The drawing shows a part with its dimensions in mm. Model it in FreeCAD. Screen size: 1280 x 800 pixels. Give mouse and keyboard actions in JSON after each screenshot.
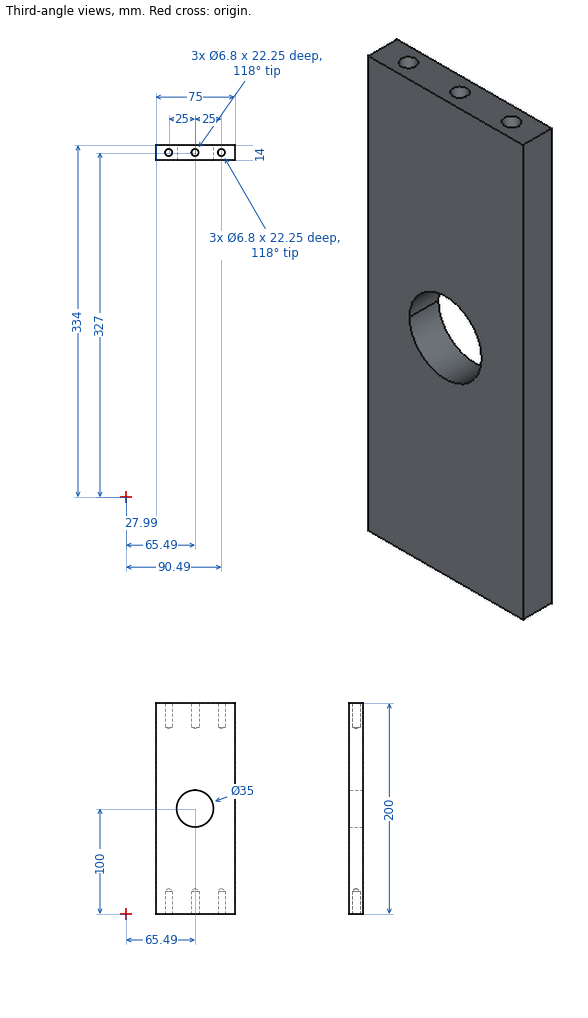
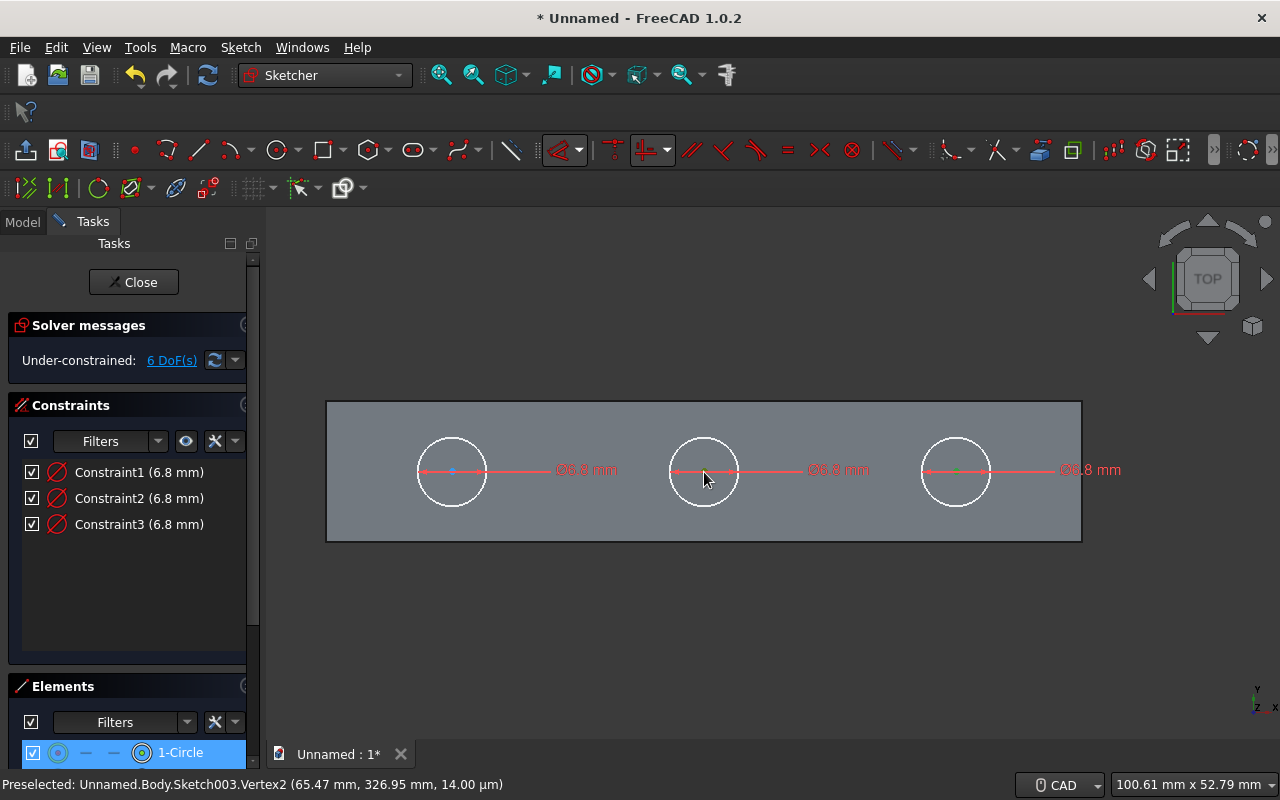
{"action": "key", "text": "h"}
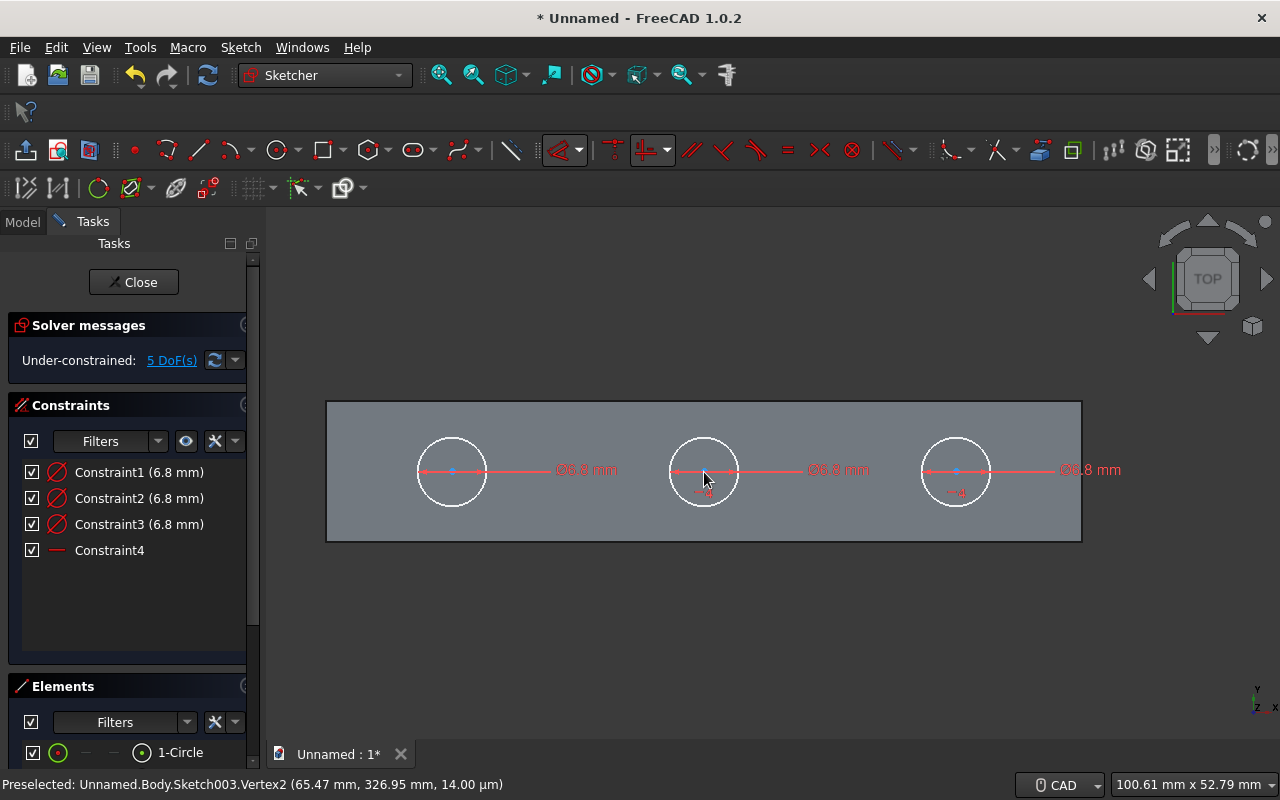
{"action": "left_click", "coordinate": [704, 472]}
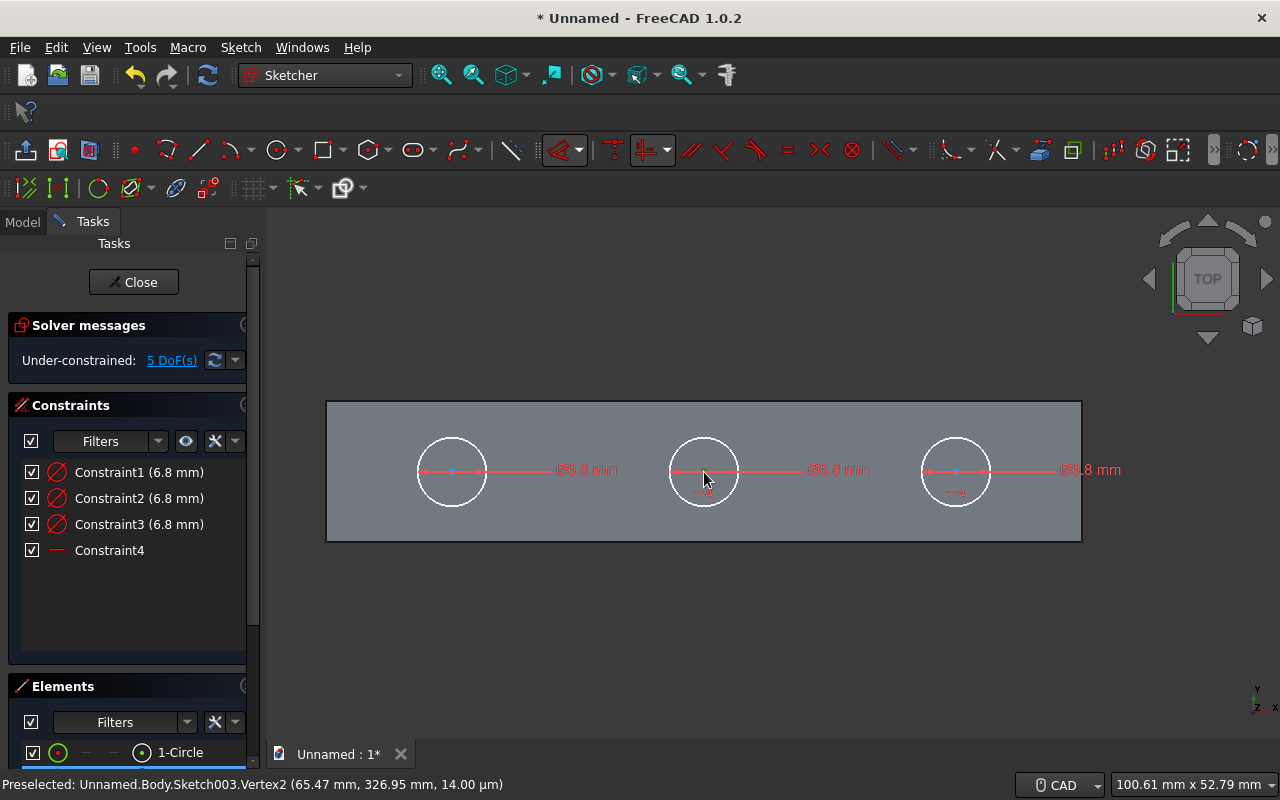
{"action": "left_click", "coordinate": [452, 472]}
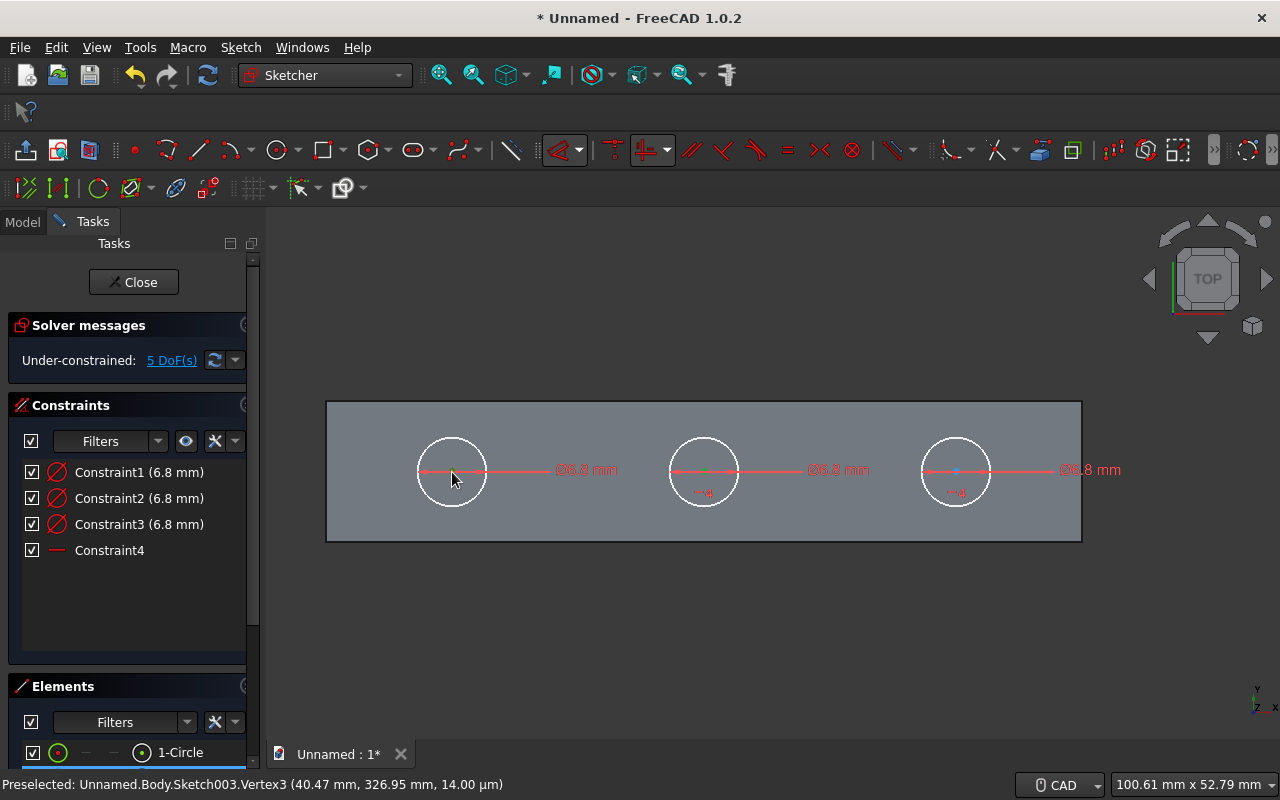
{"action": "left_click", "coordinate": [670, 150]}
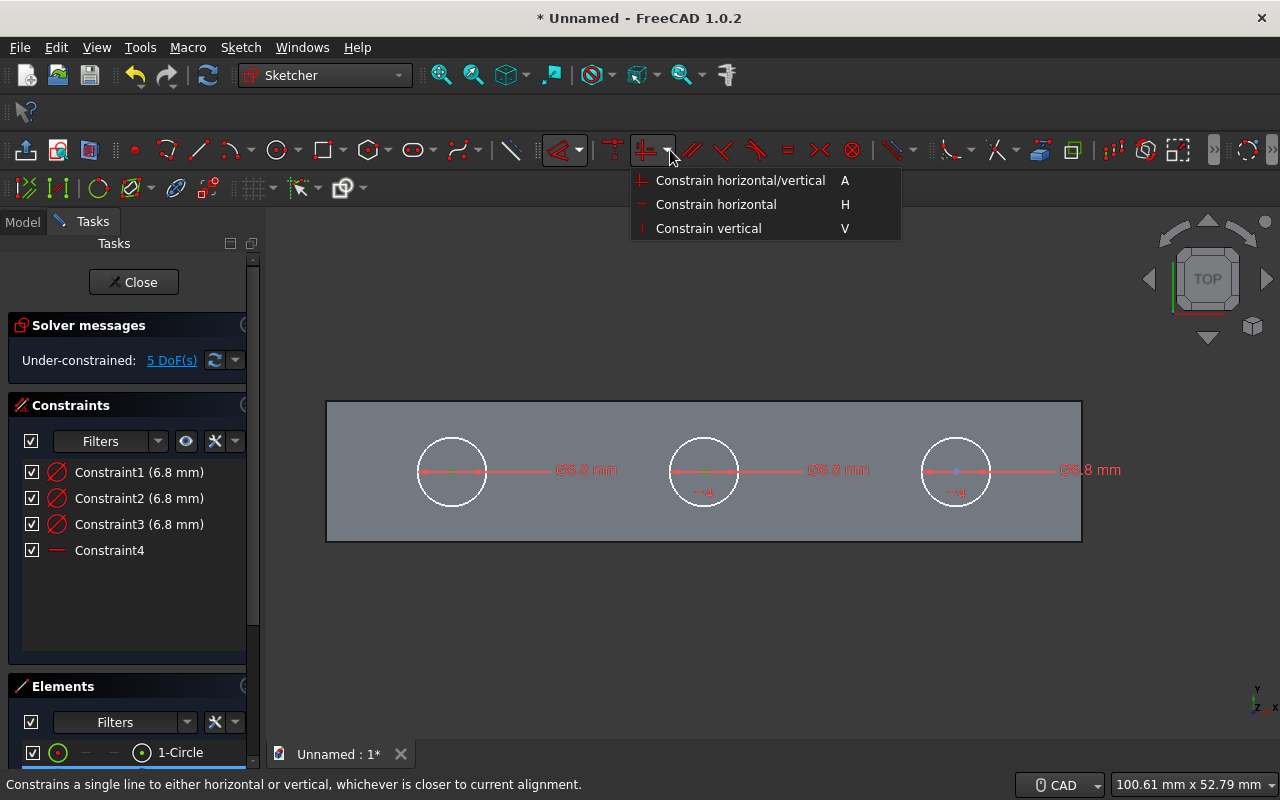
{"action": "left_click", "coordinate": [766, 204]}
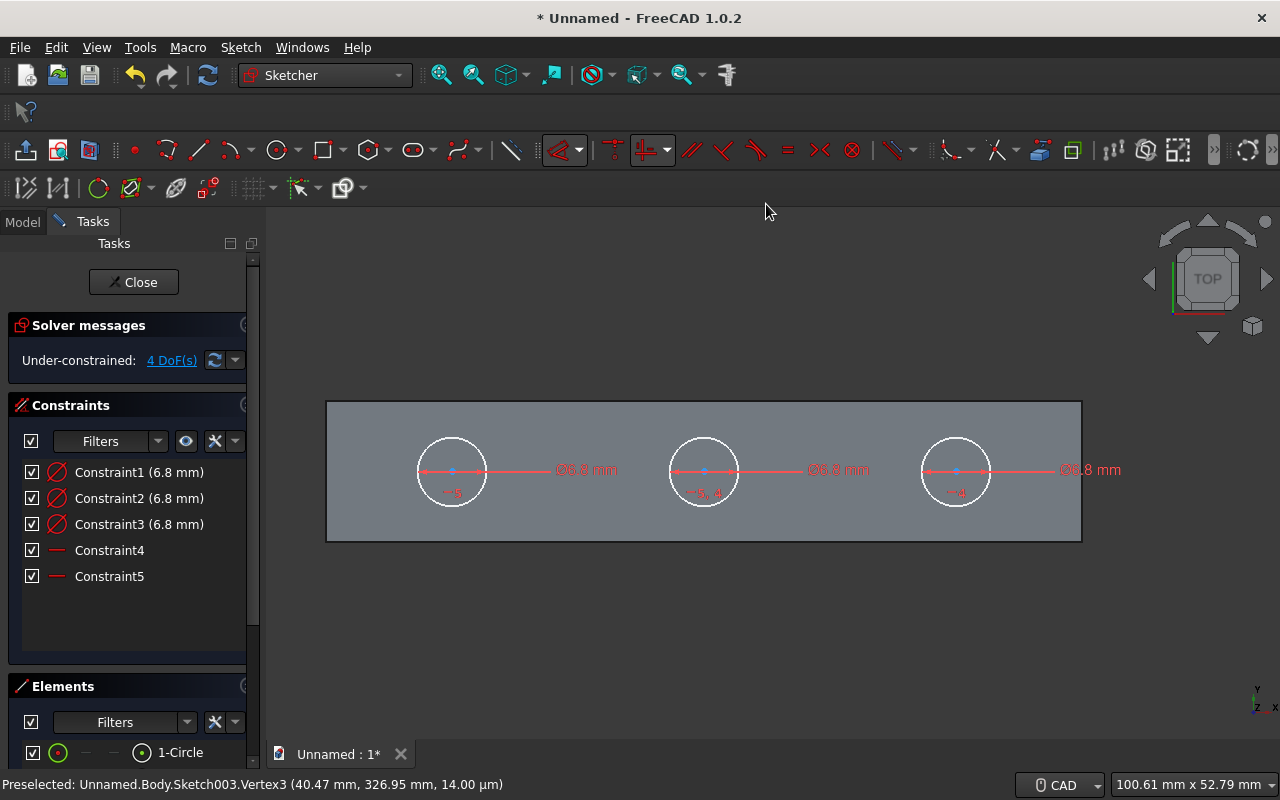
{"action": "left_click", "coordinate": [956, 472]}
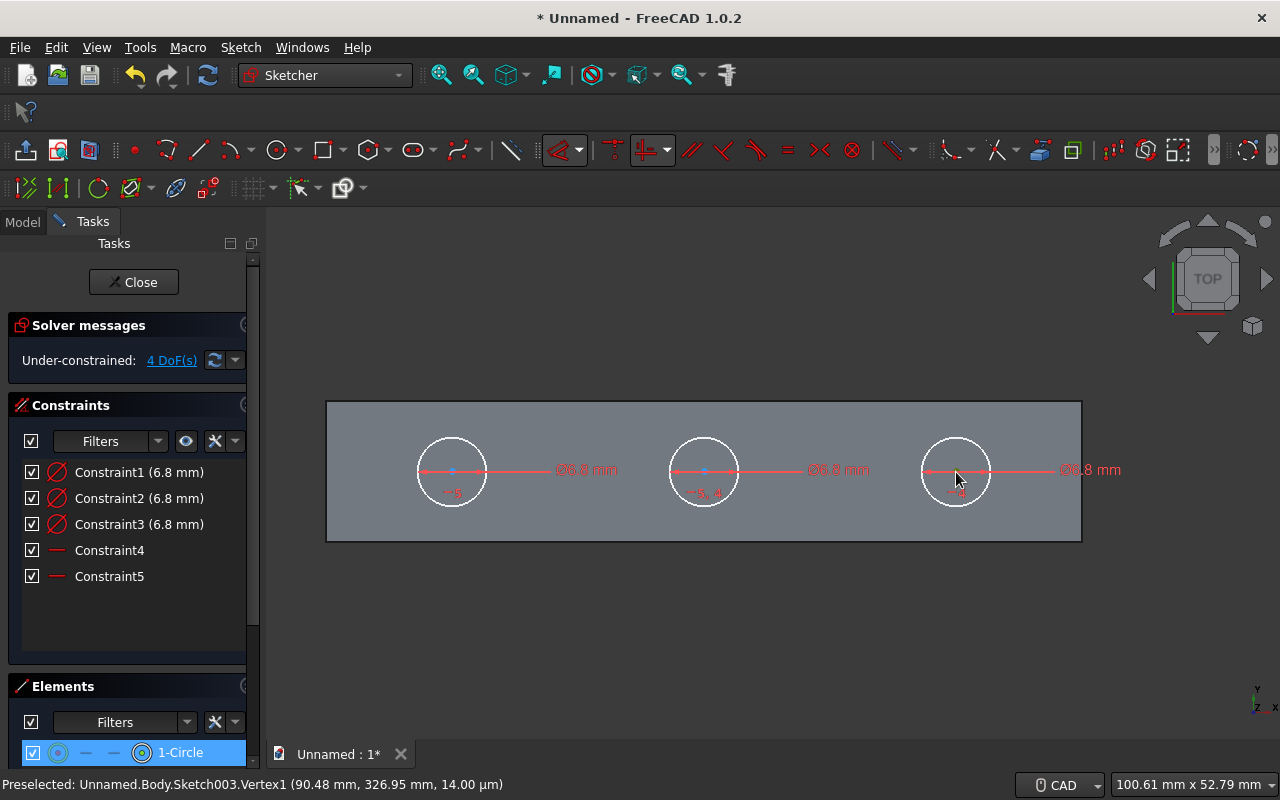
{"action": "left_click", "coordinate": [582, 150]}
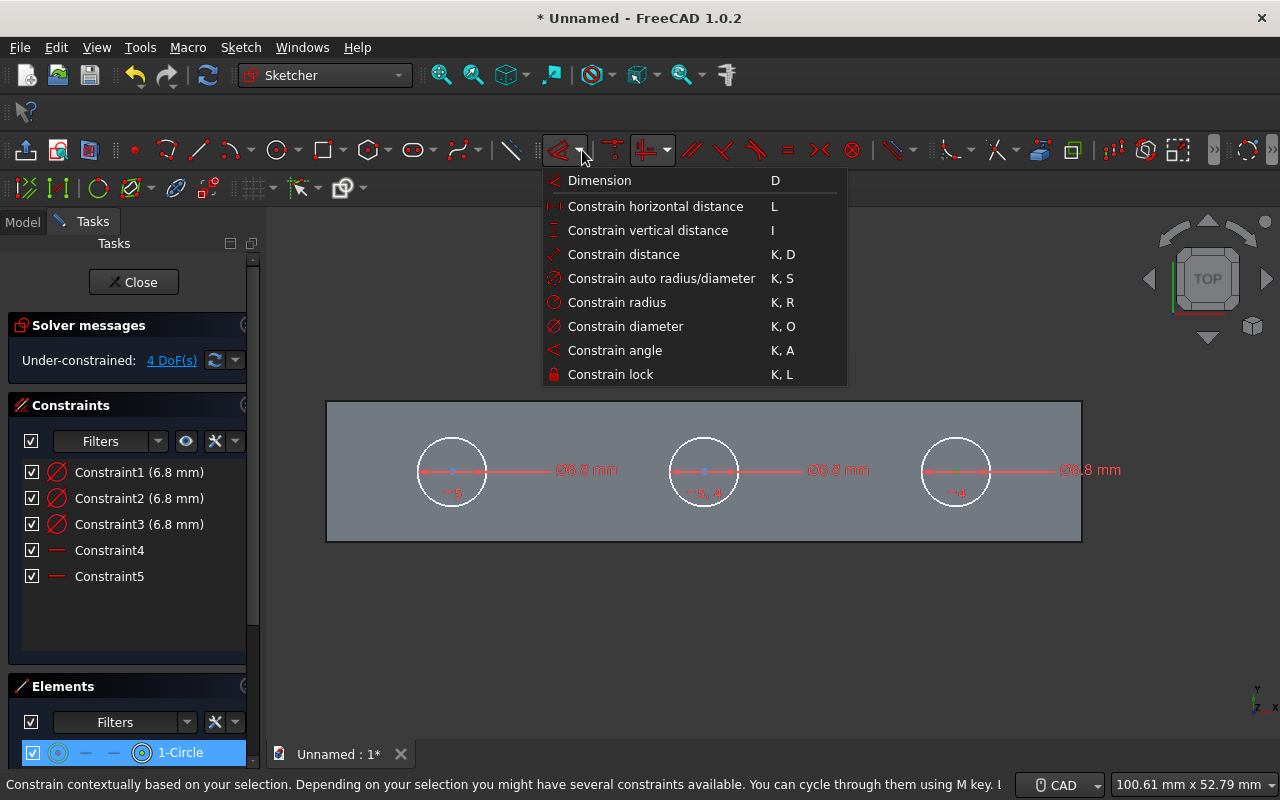
{"action": "left_click", "coordinate": [695, 230]}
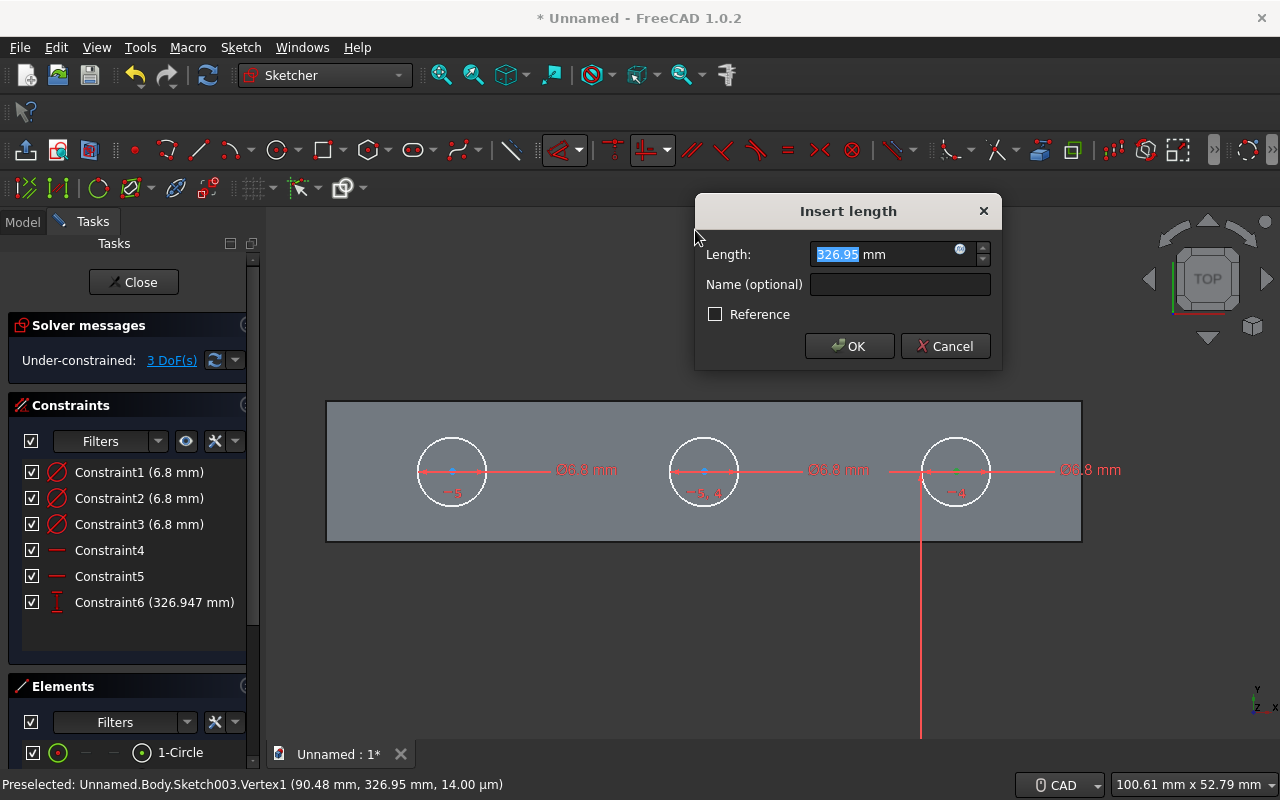
{"action": "type", "text": "327"}
{"action": "key", "text": "Return"}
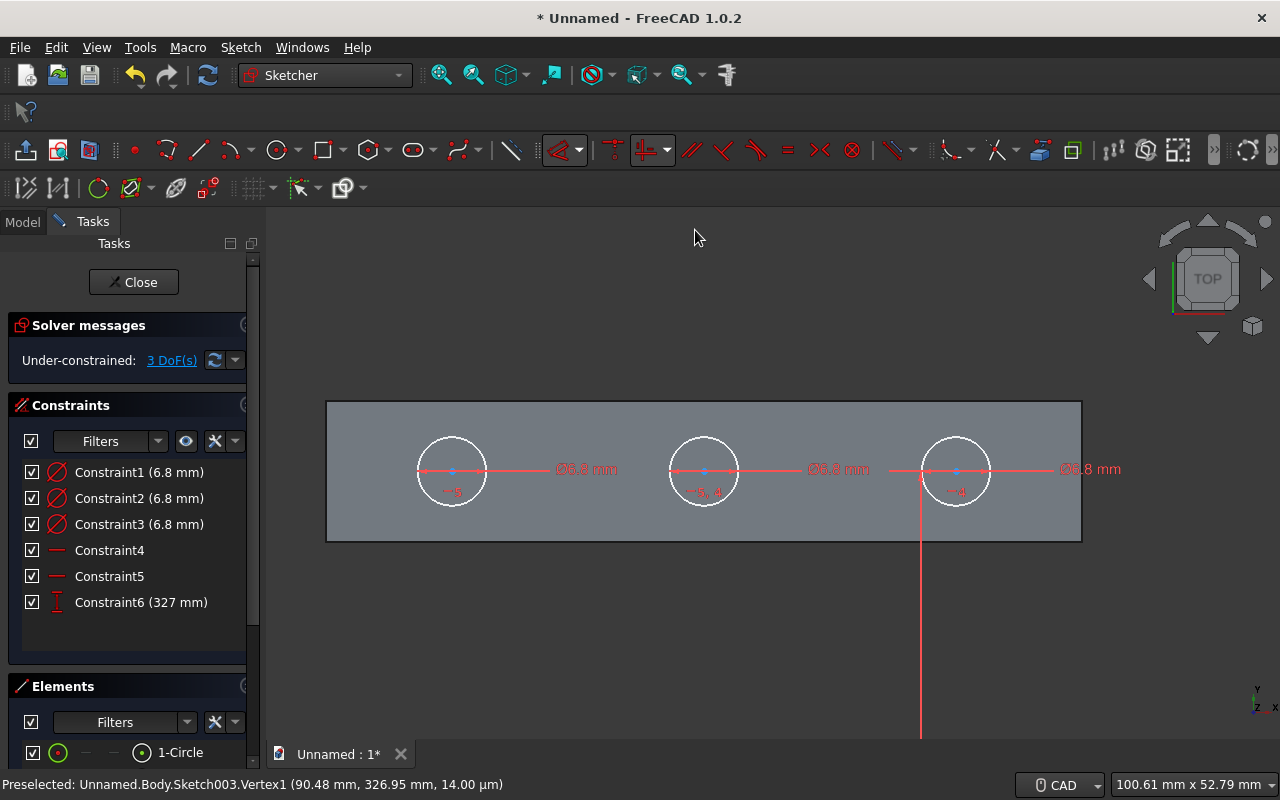
{"action": "left_click", "coordinate": [956, 471]}